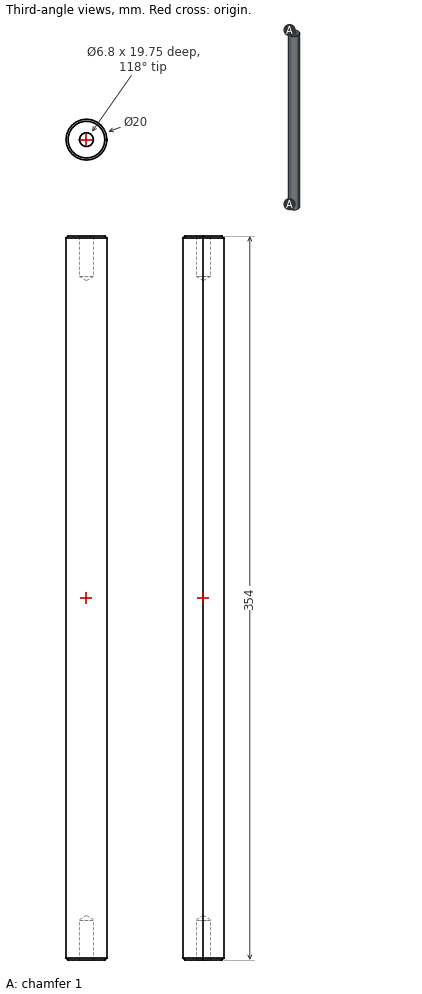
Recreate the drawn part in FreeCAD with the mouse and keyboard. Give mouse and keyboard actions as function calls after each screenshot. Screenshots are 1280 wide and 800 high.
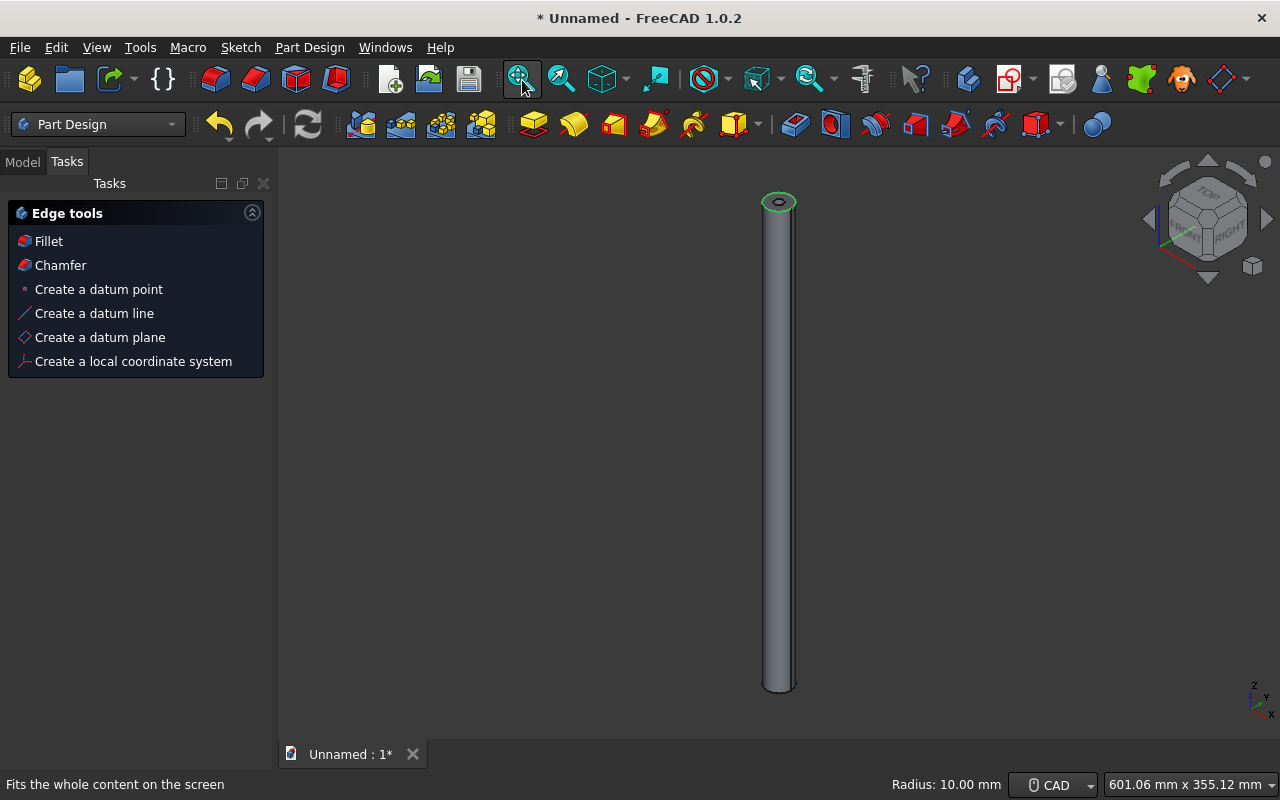
key(1)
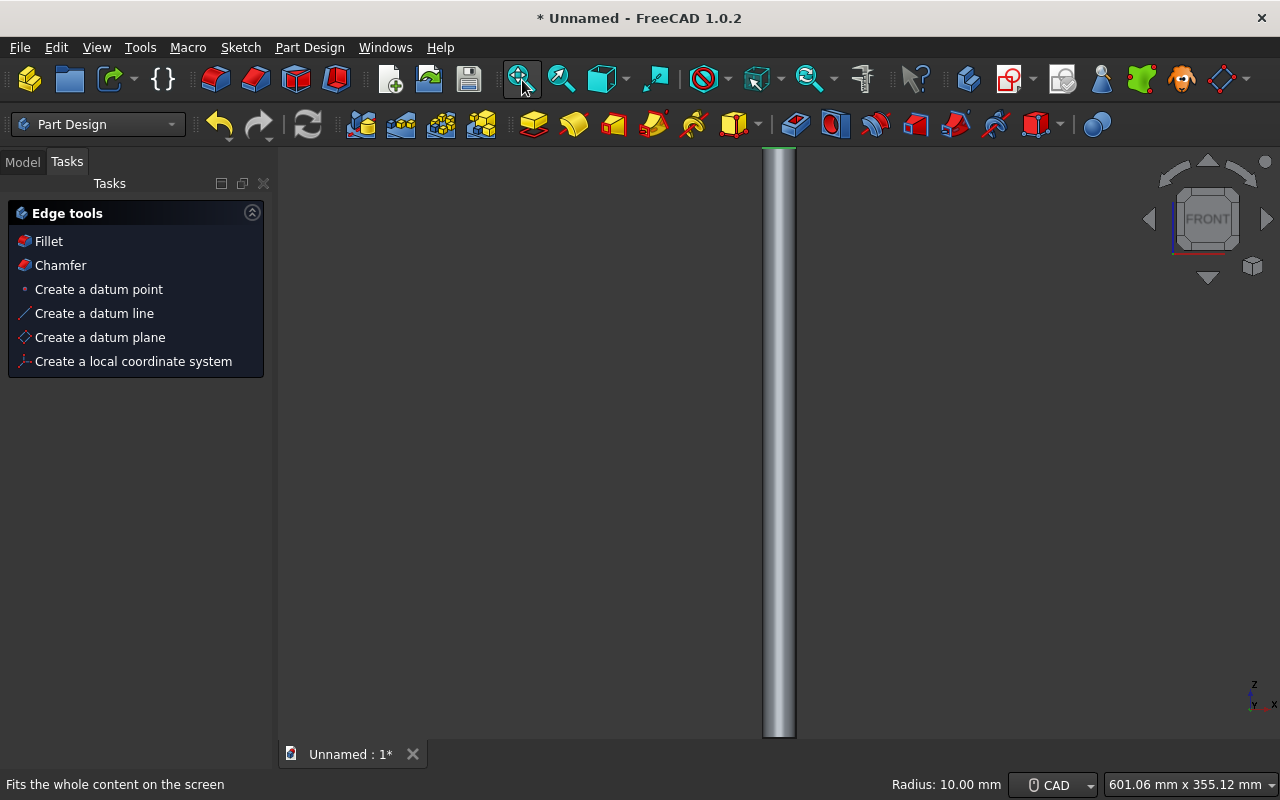
key(3)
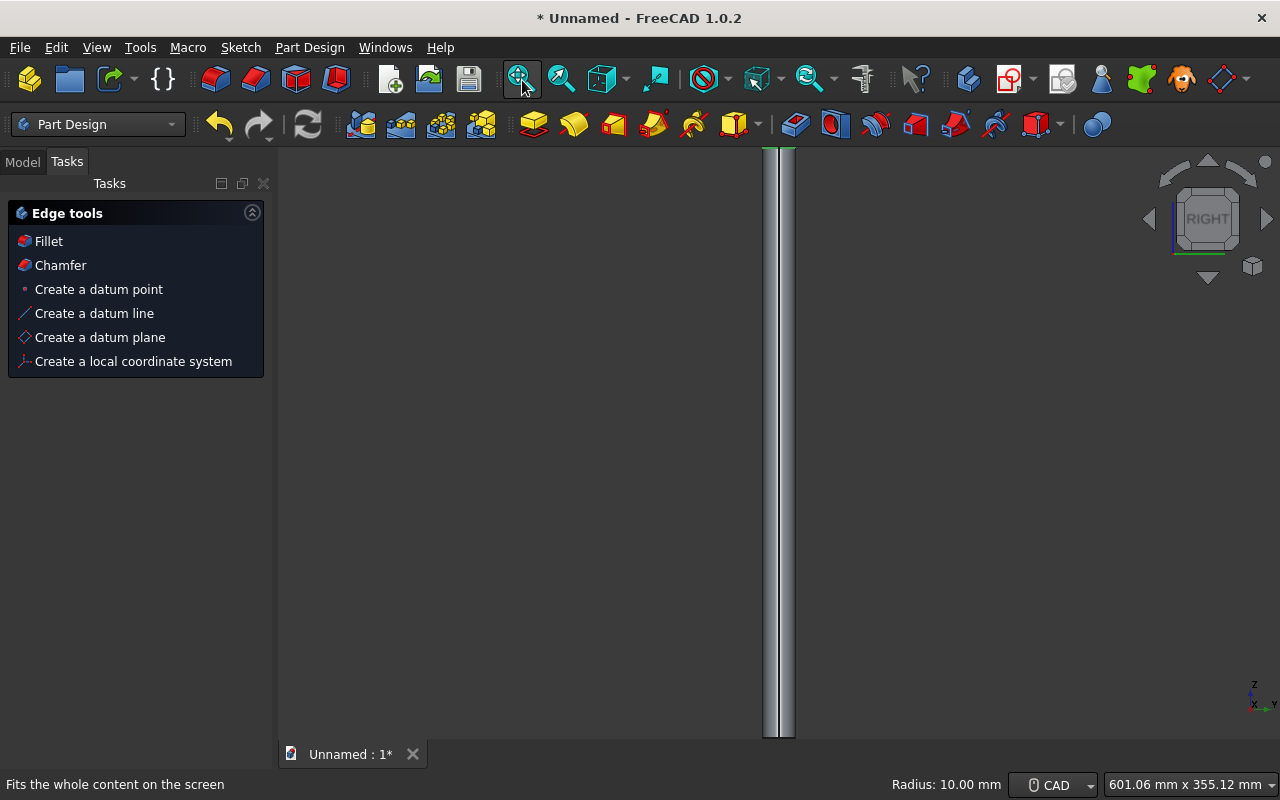
key(5)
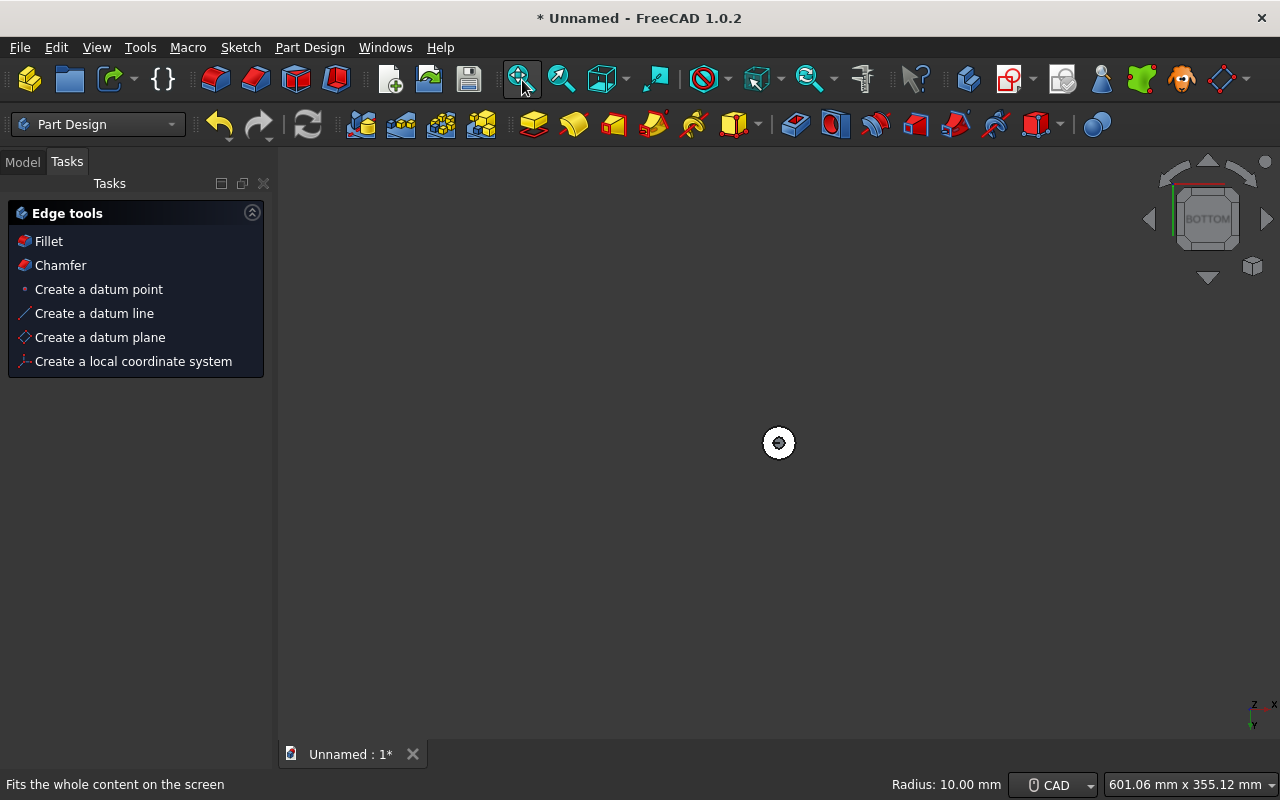
key(v)
key(f)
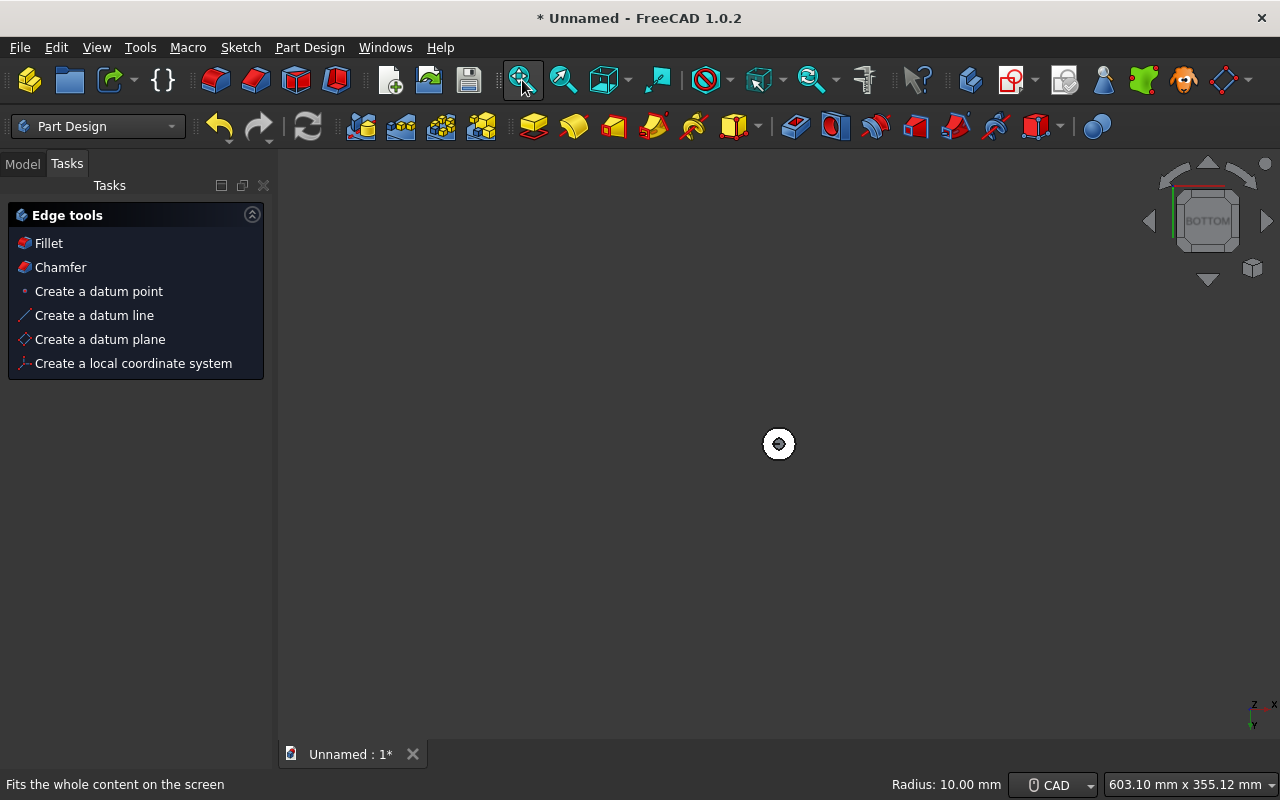
click(762, 443, ctrl)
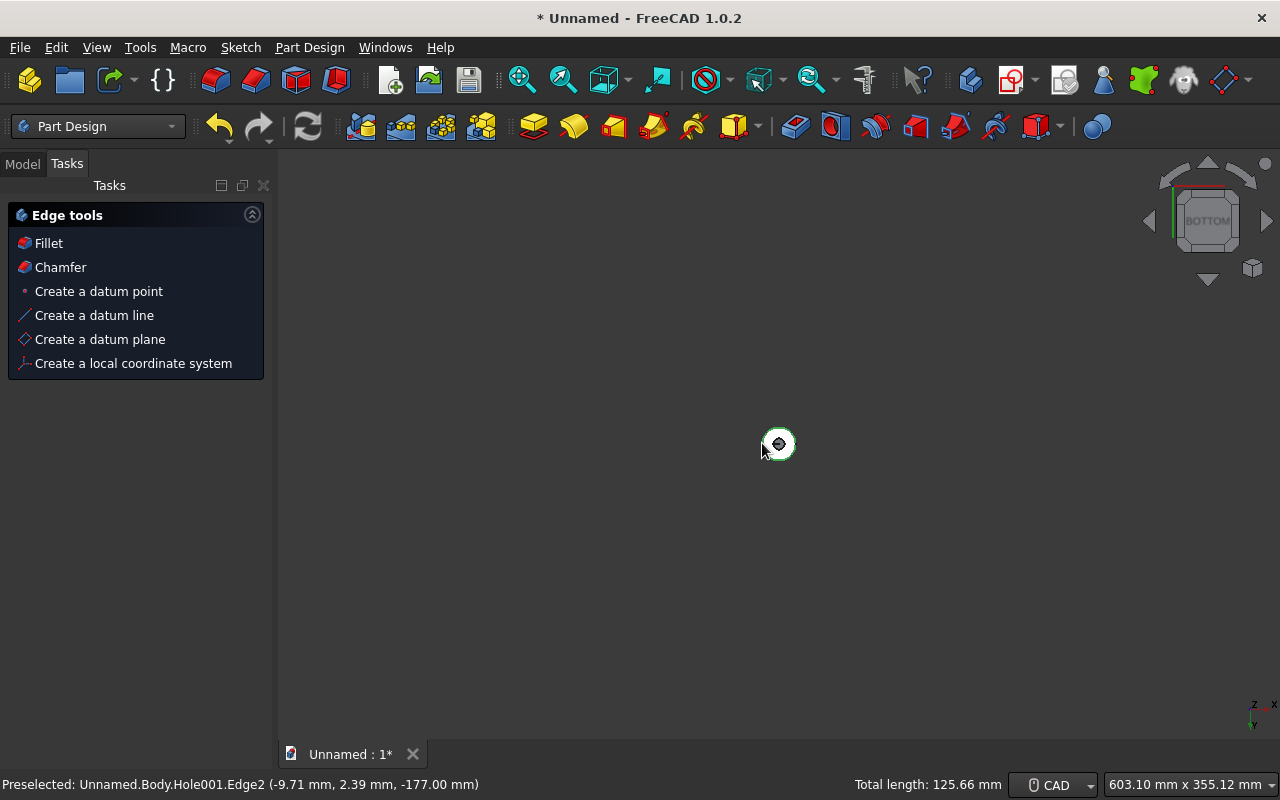
click(256, 80)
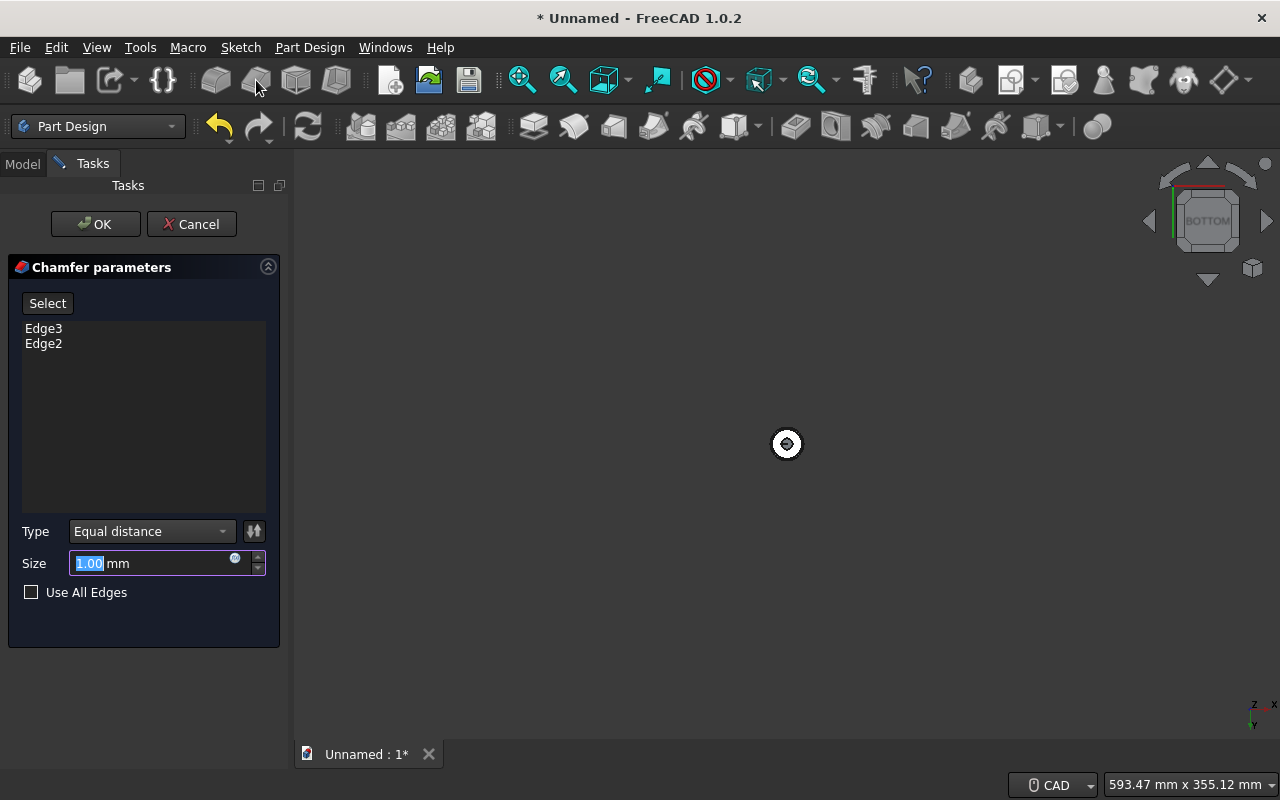
text(1)
key(Tab)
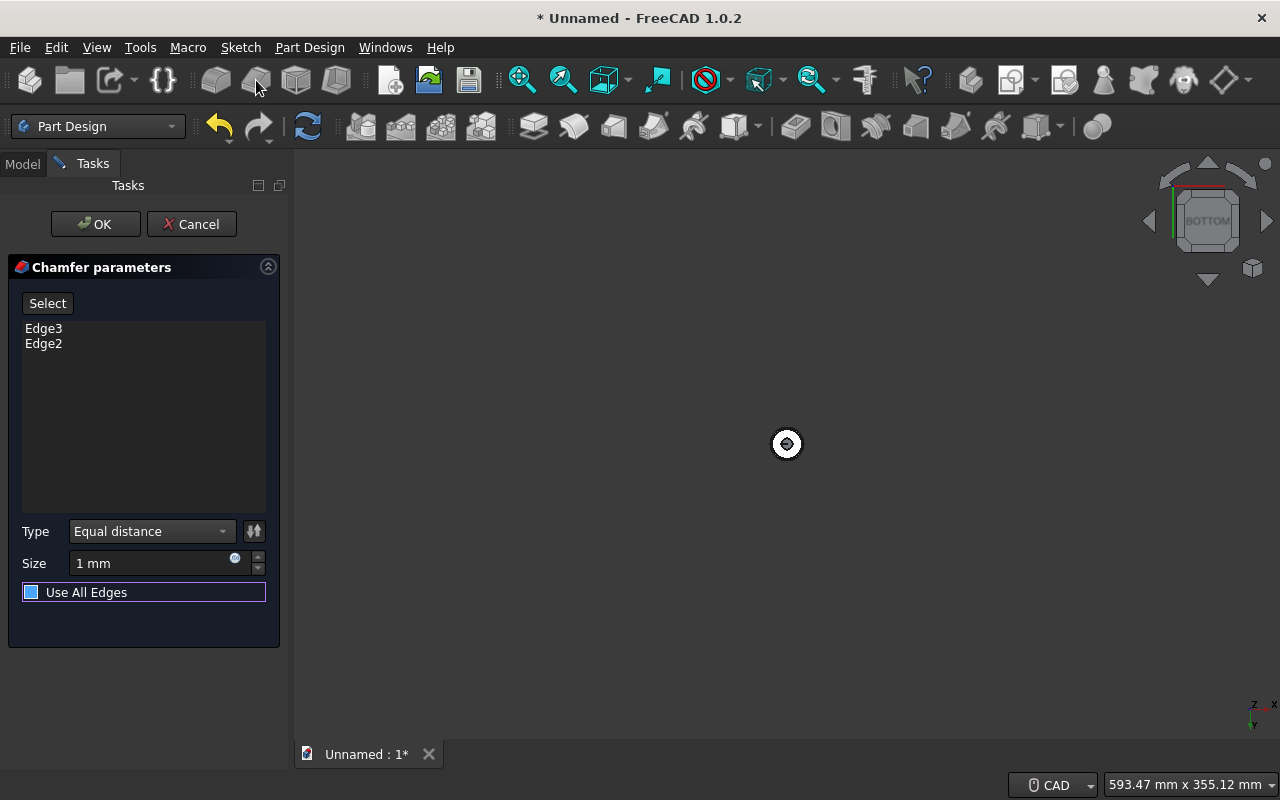
click(96, 224)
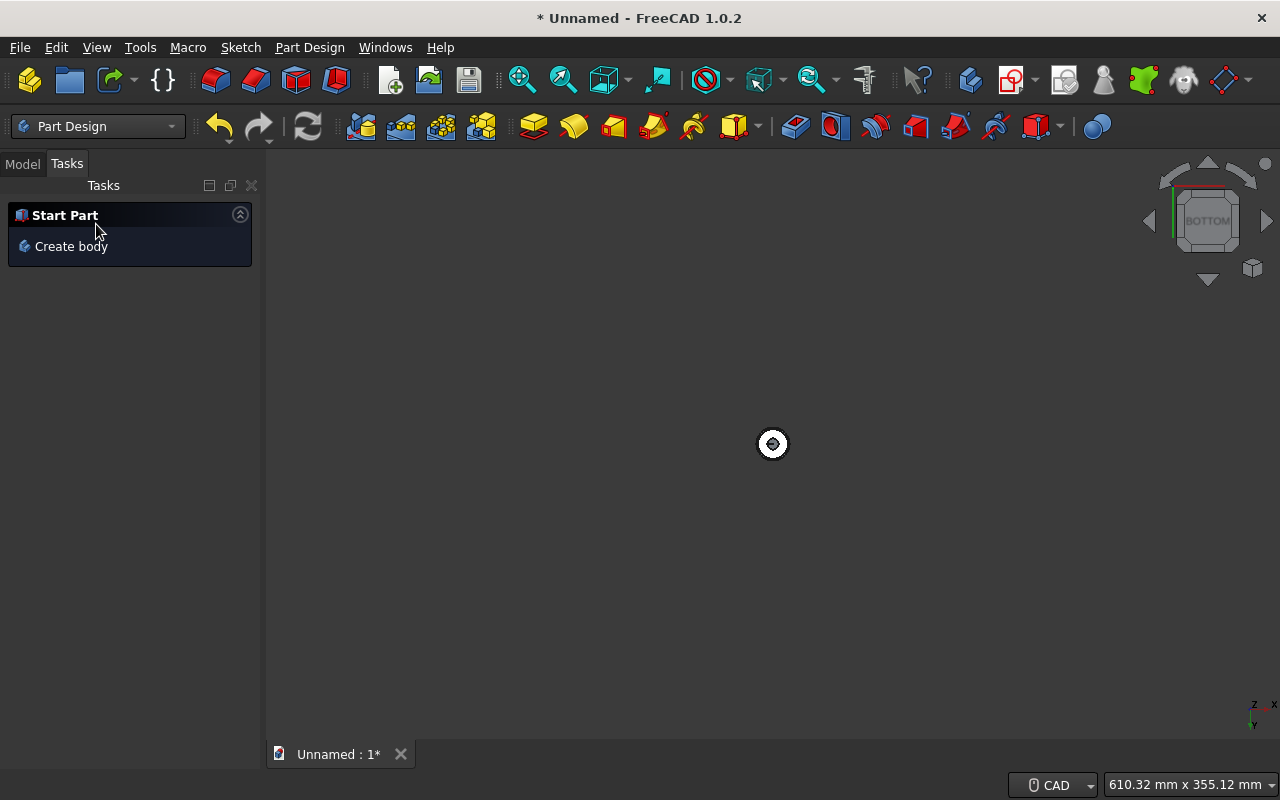
key(0)